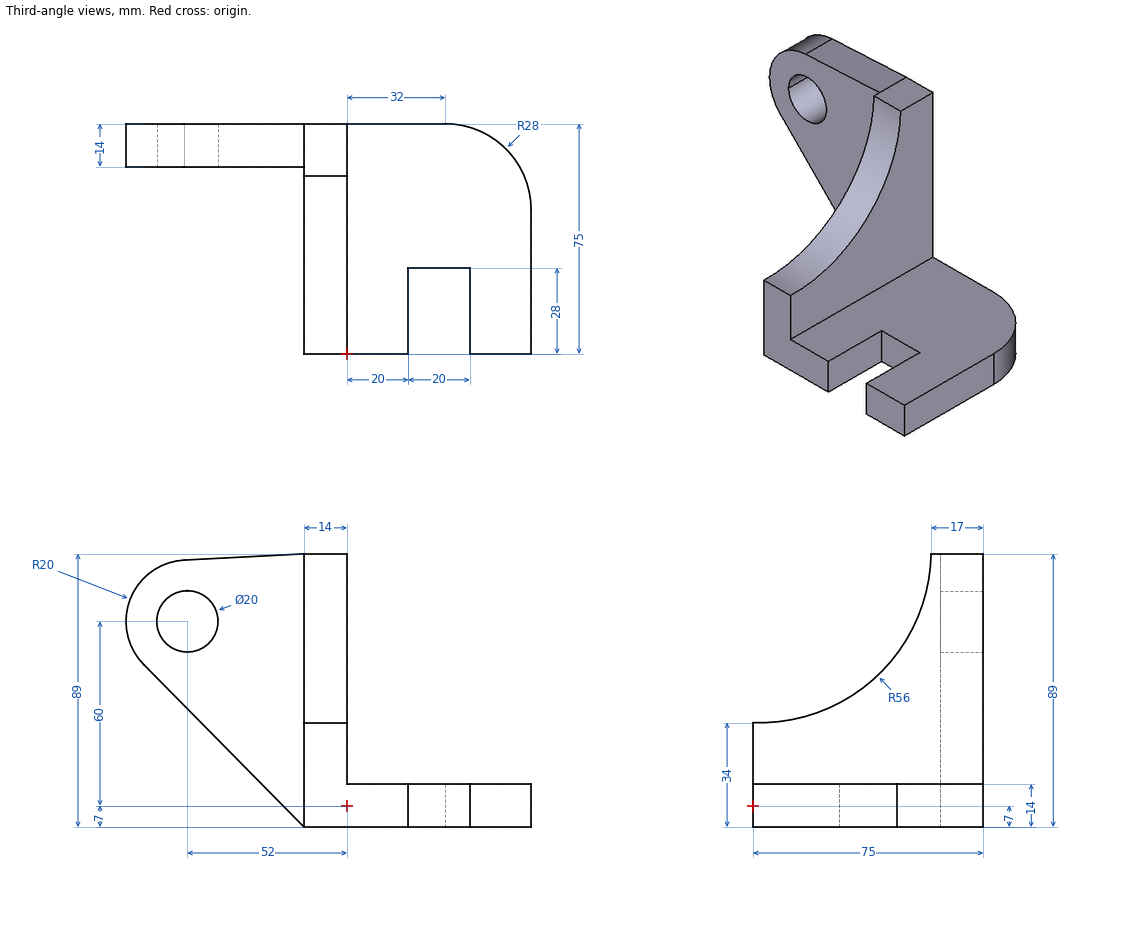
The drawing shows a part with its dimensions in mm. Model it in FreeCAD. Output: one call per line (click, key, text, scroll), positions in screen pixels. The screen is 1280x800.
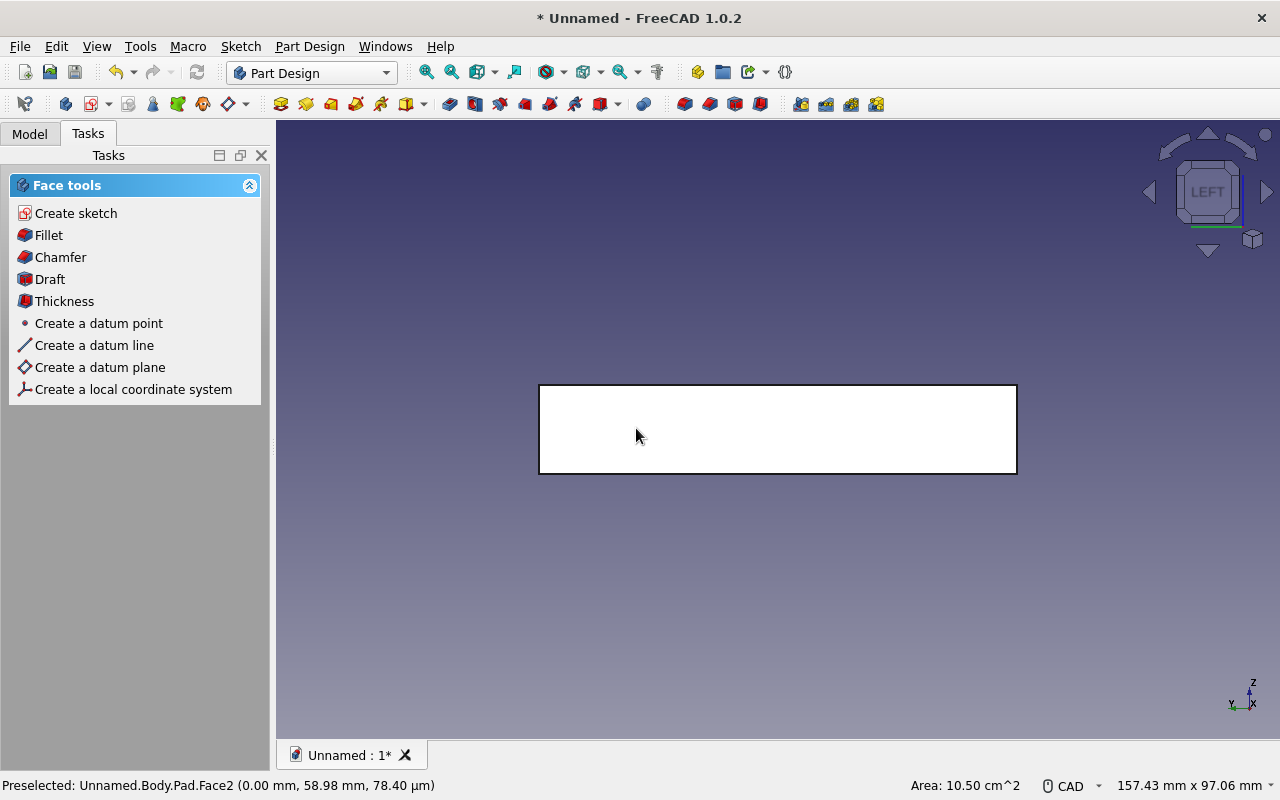
click(90, 104)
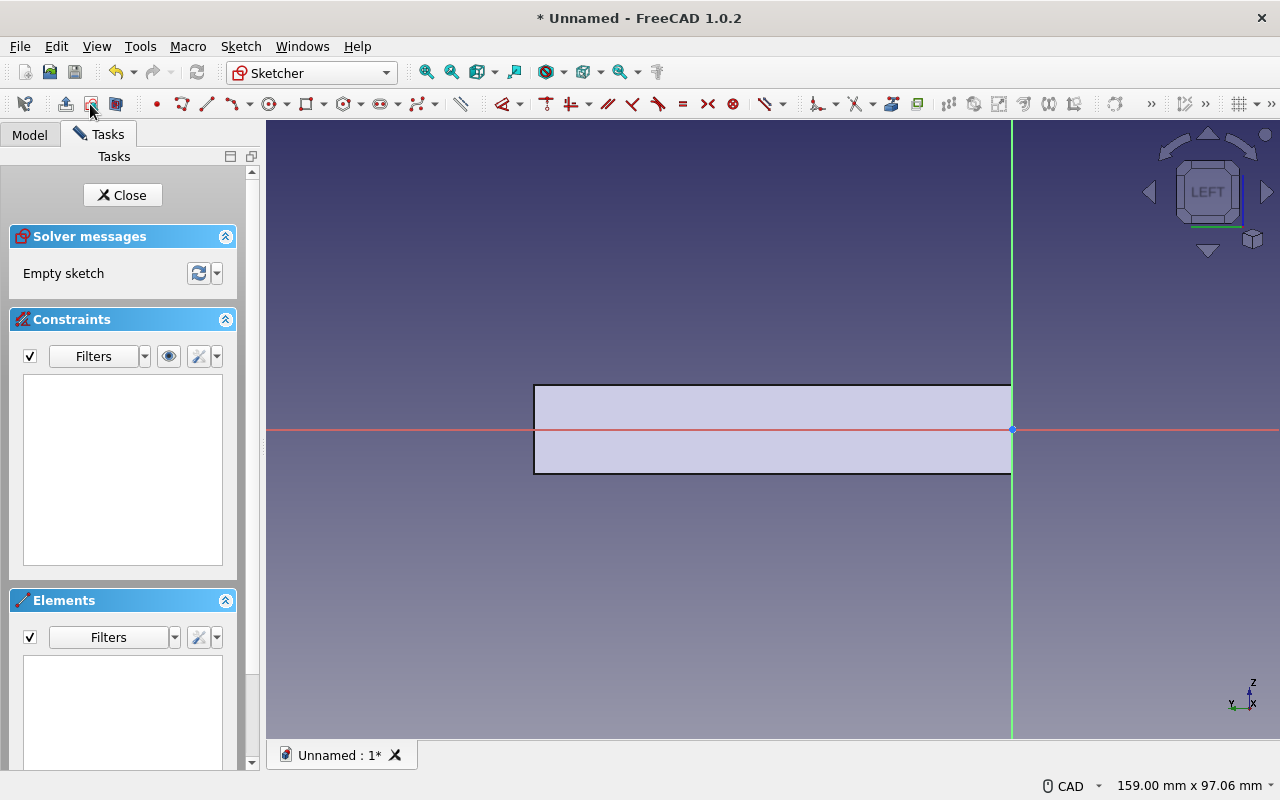
scroll(621, 711, down, 3)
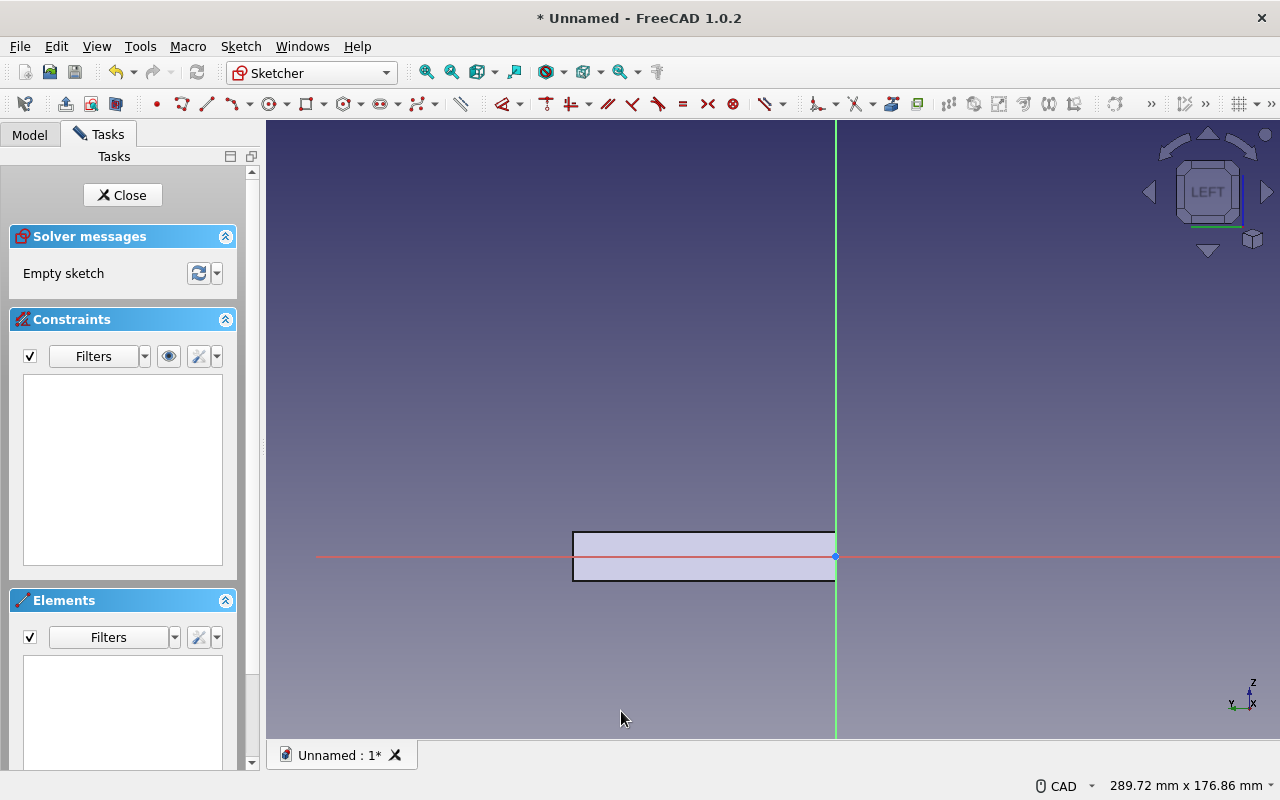
click(182, 104)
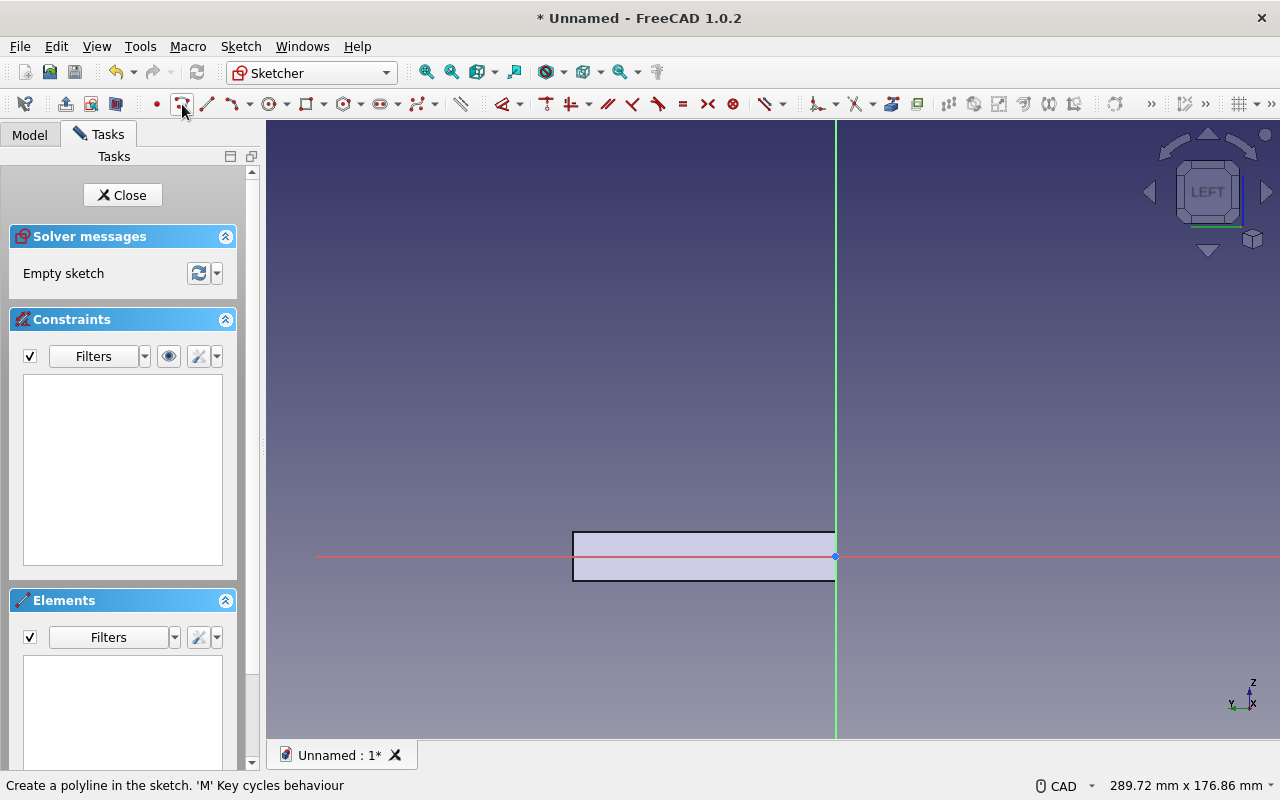
click(633, 270)
click(573, 270)
click(573, 581)
click(836, 581)
click(827, 462)
right_click(827, 462)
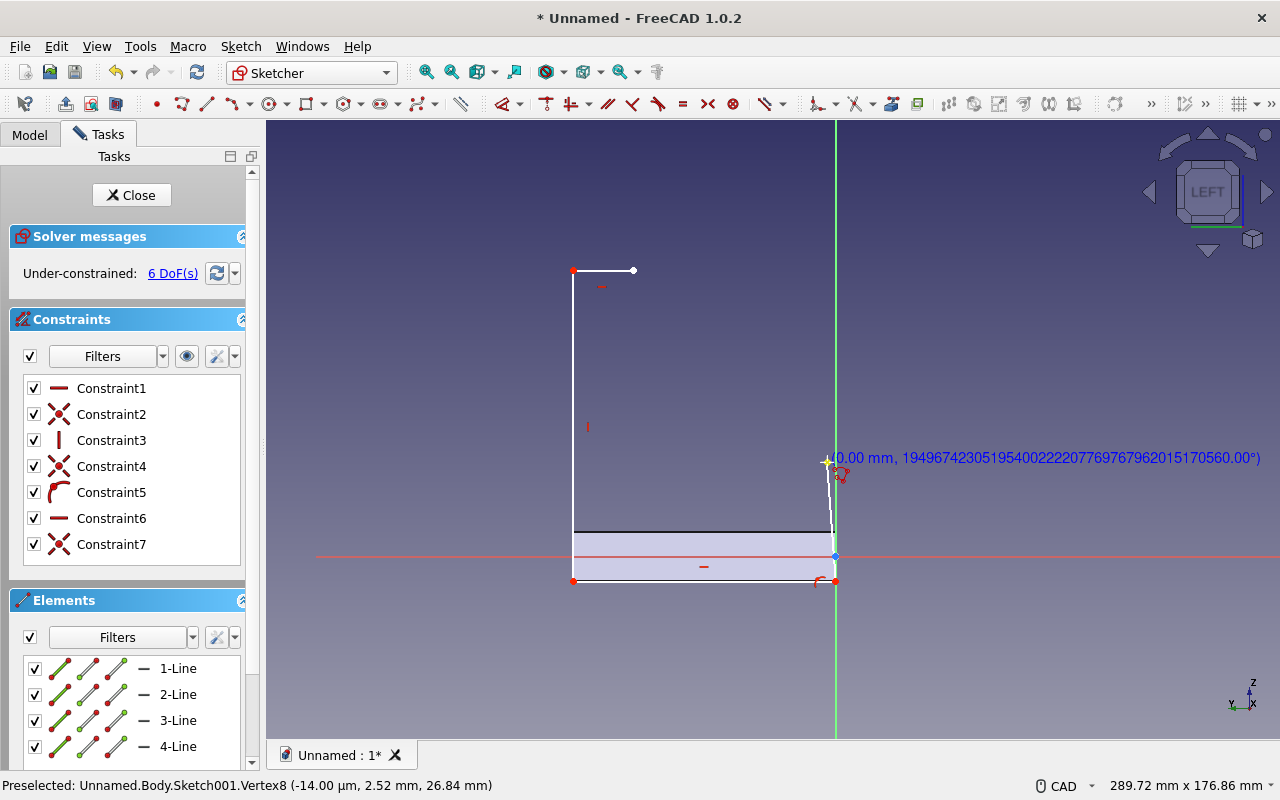
click(232, 104)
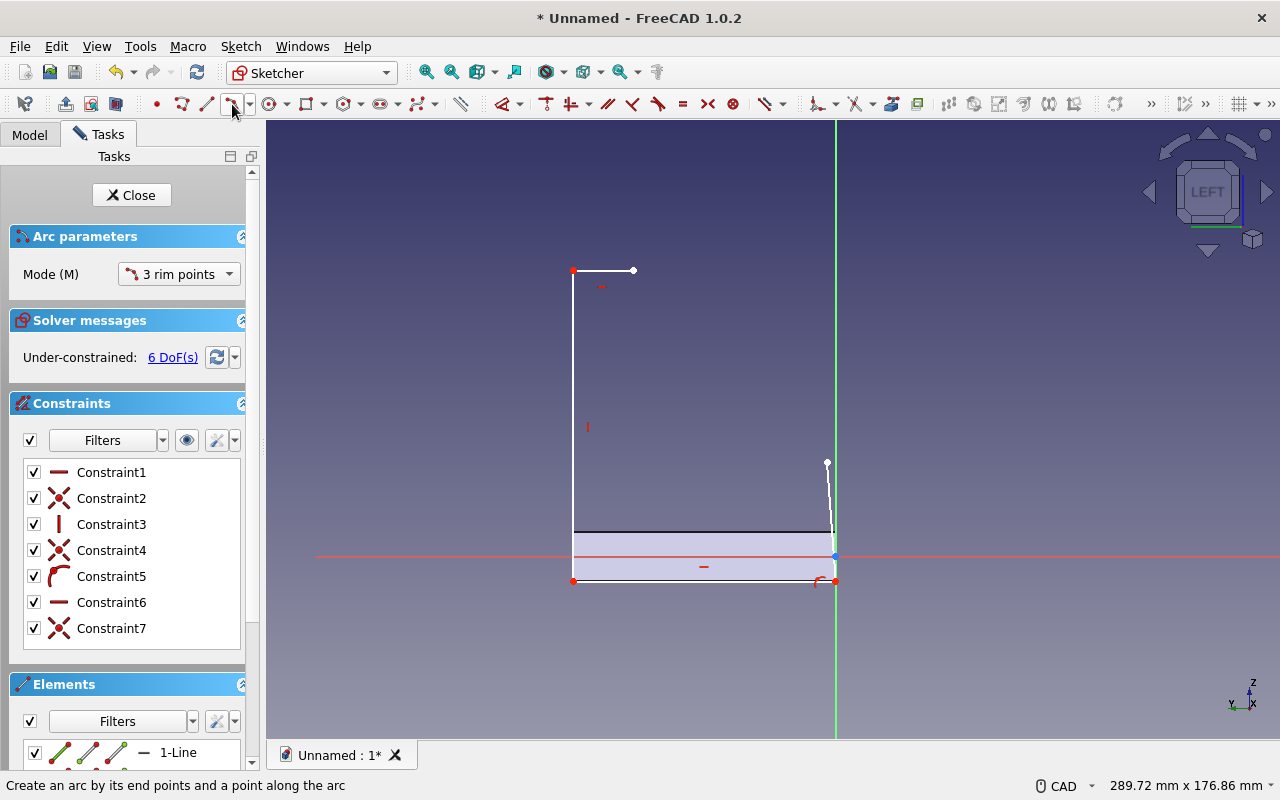
click(827, 463)
click(633, 271)
click(694, 409)
key(Escape)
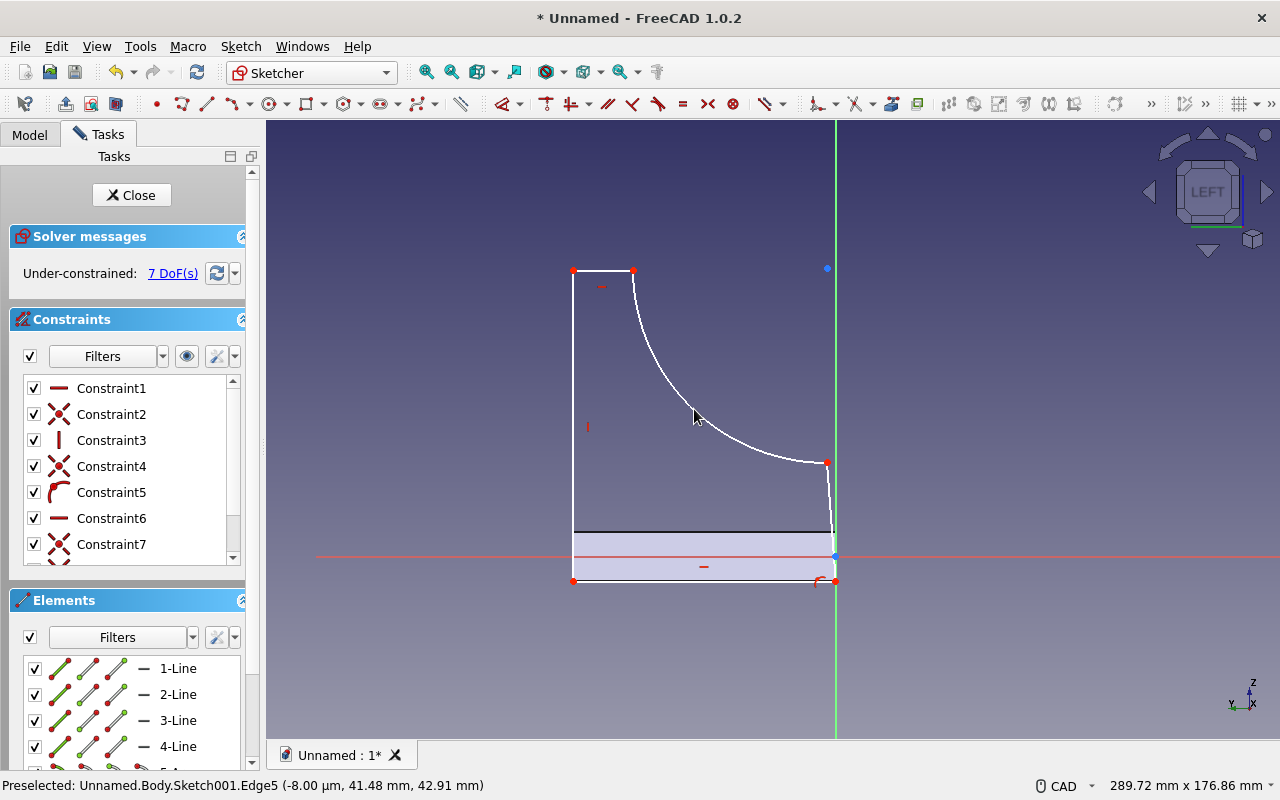
scroll(833, 546, up, 2)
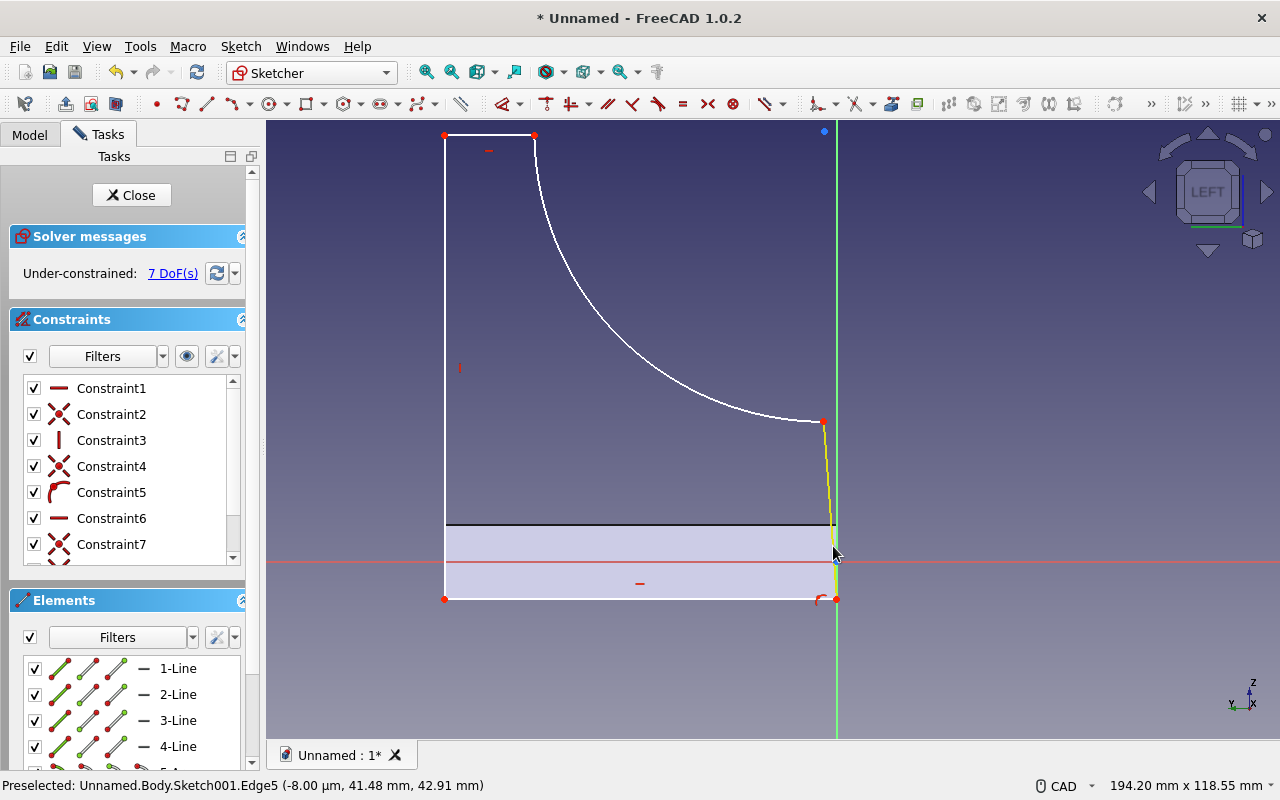
click(833, 546)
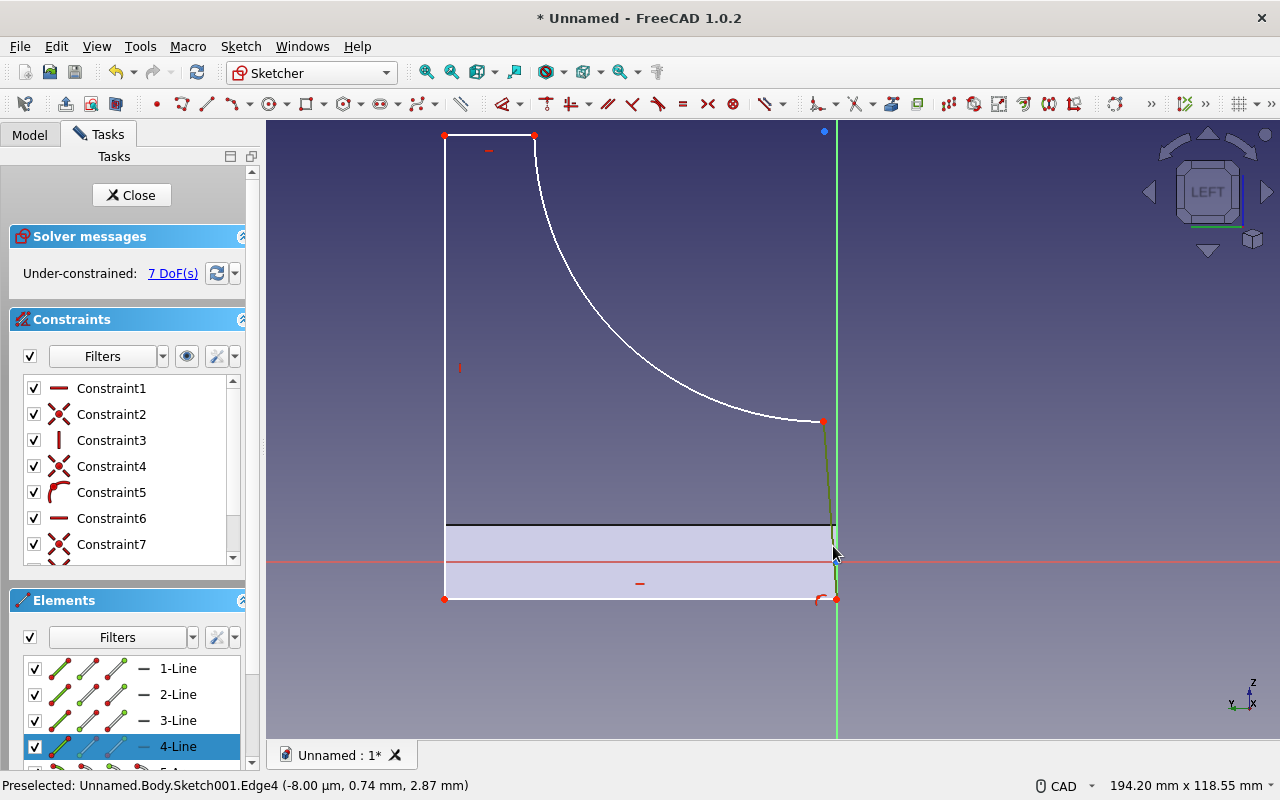
key(v)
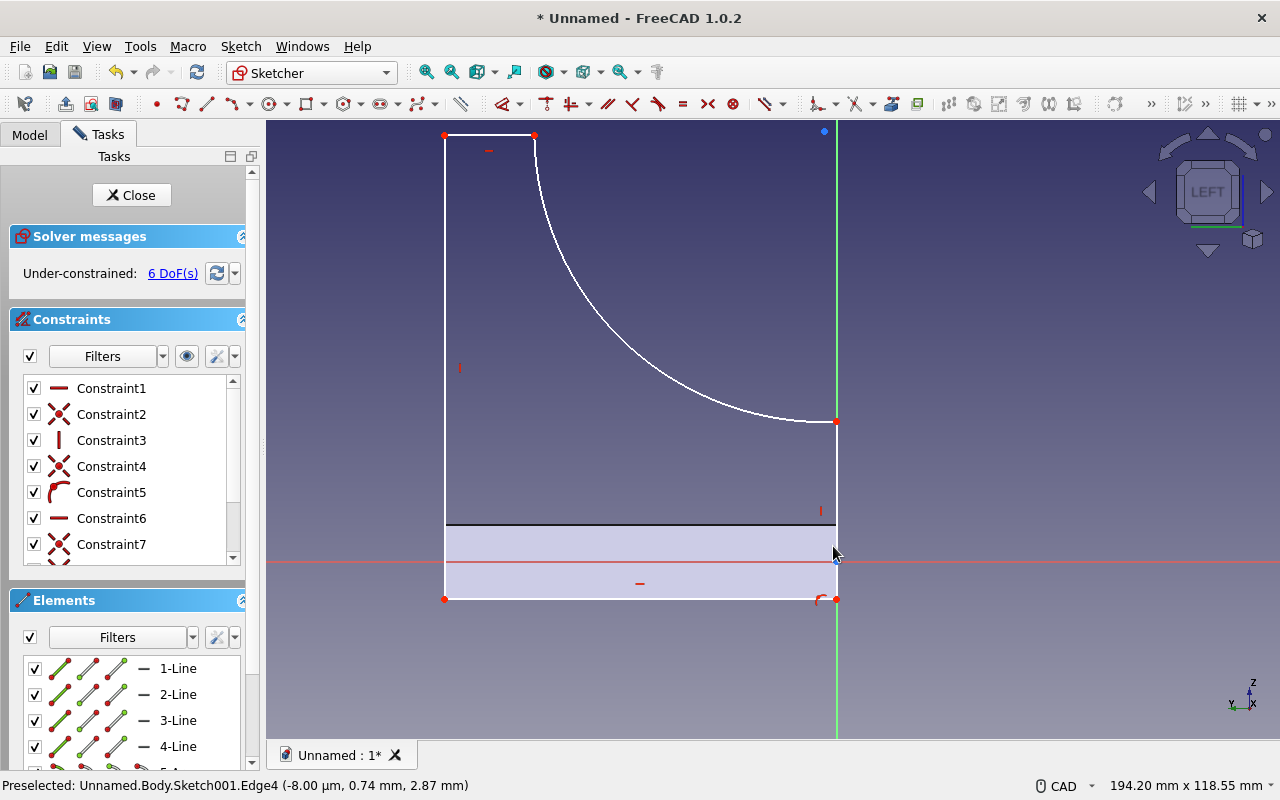
click(502, 104)